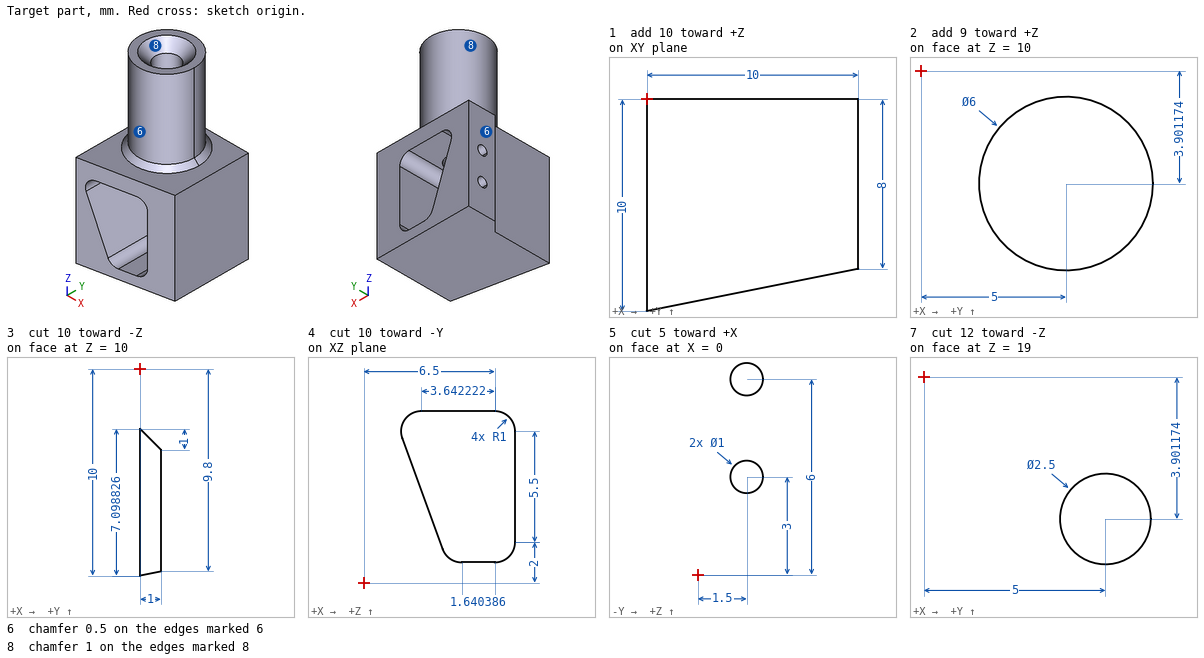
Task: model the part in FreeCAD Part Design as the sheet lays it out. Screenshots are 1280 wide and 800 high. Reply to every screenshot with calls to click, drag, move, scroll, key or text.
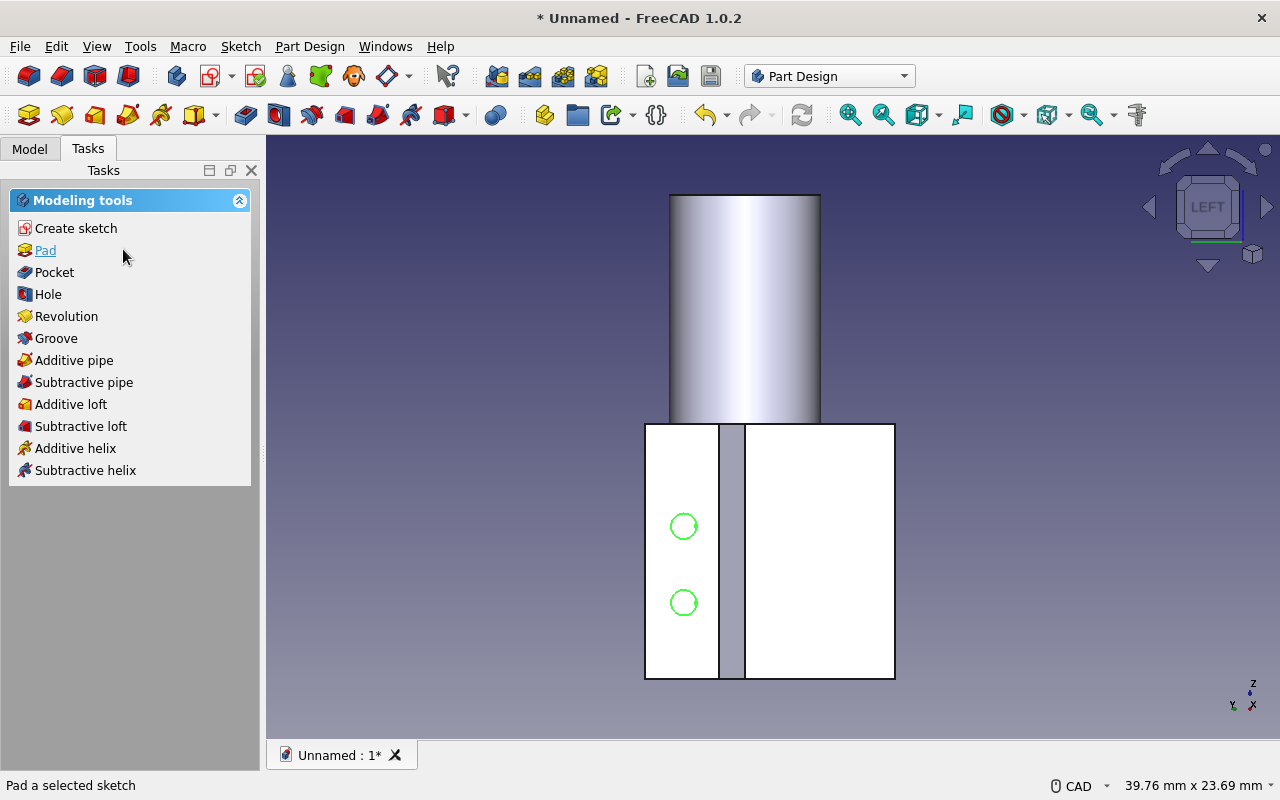
click(246, 116)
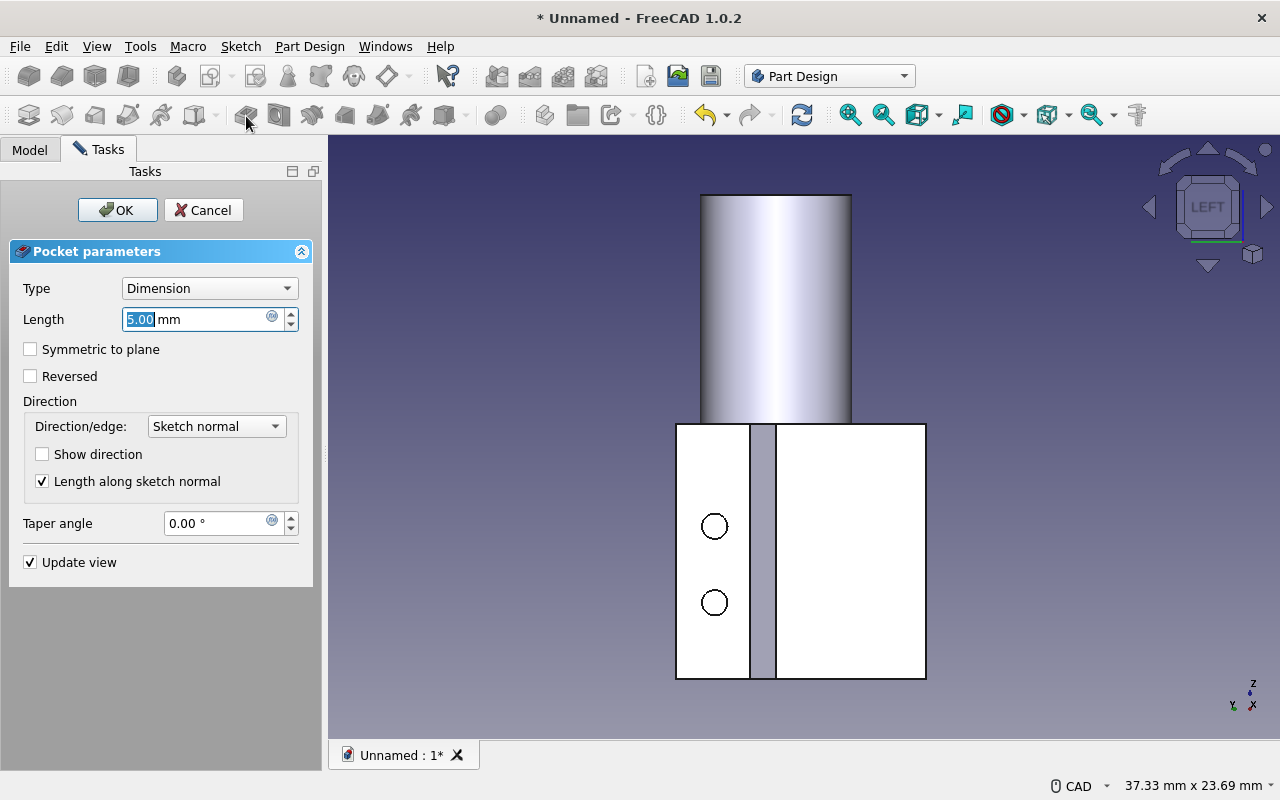
text(5)
key(Tab)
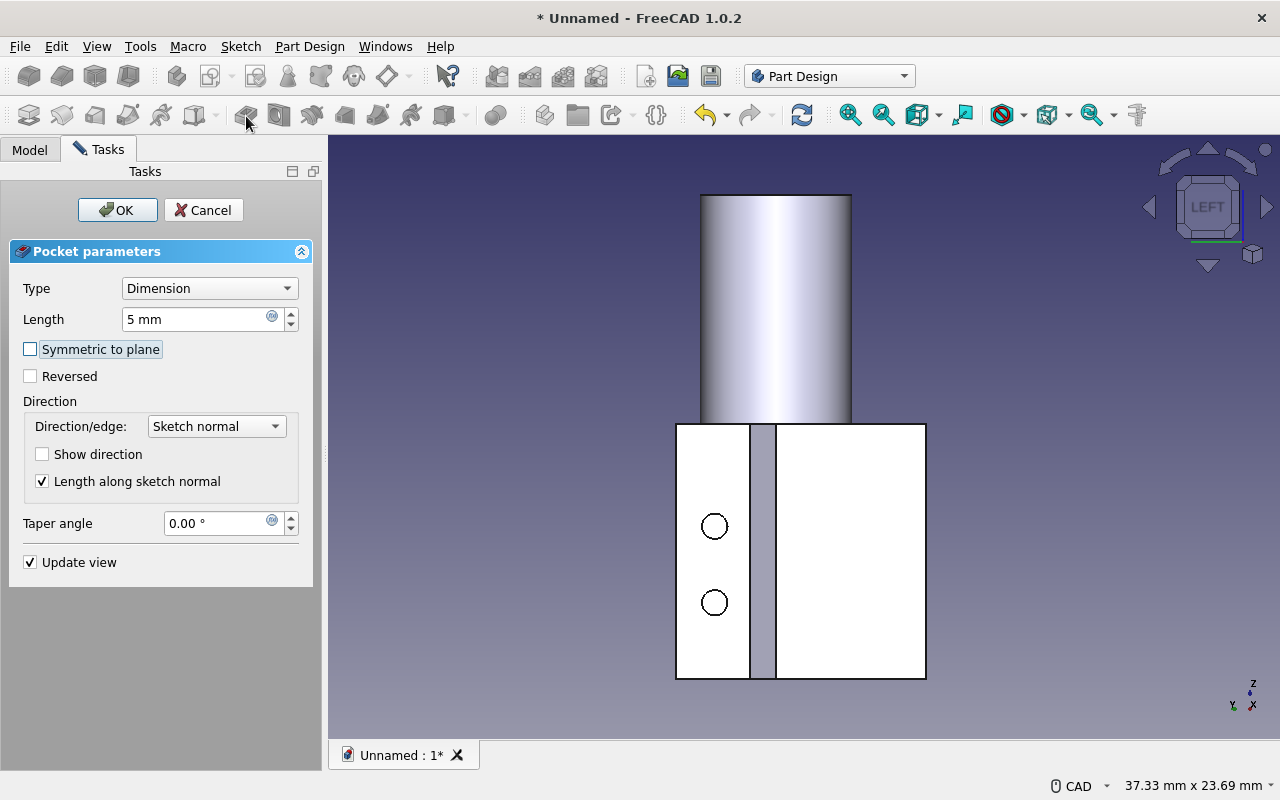
click(118, 210)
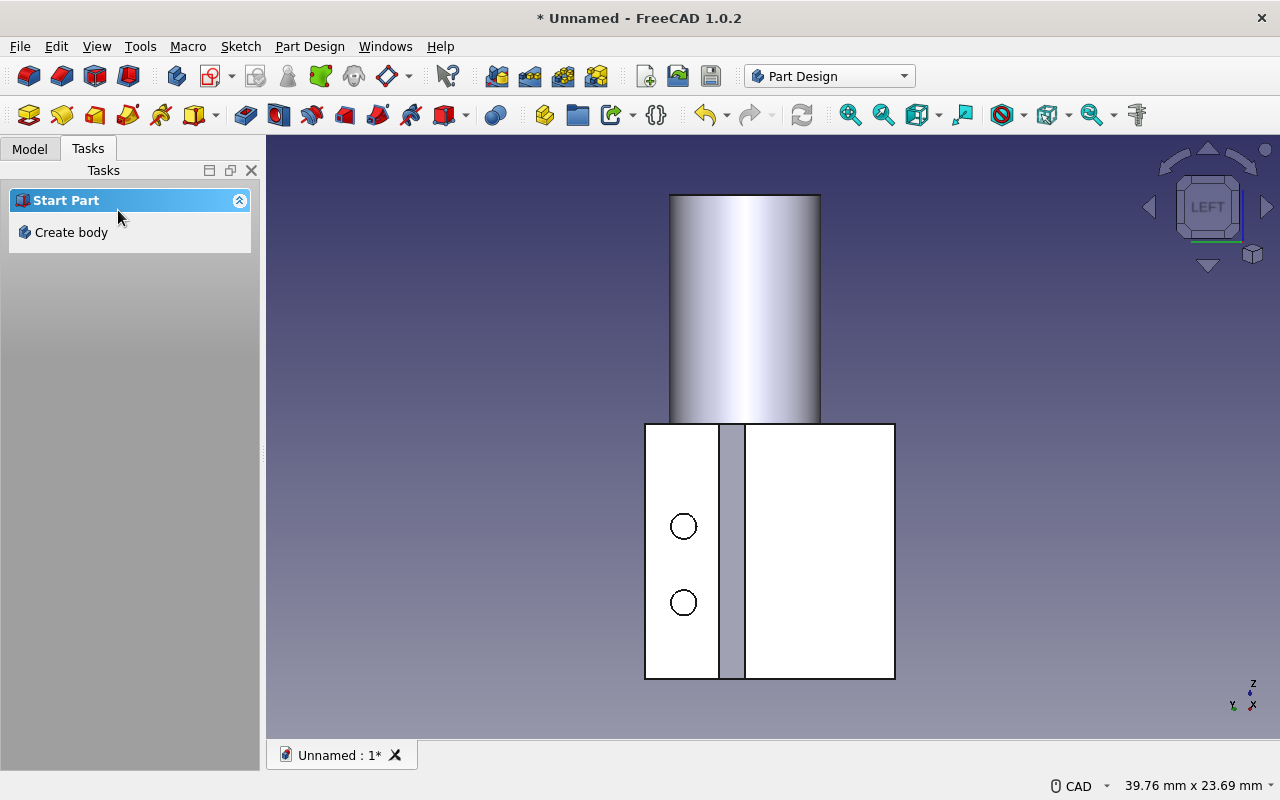
key(0)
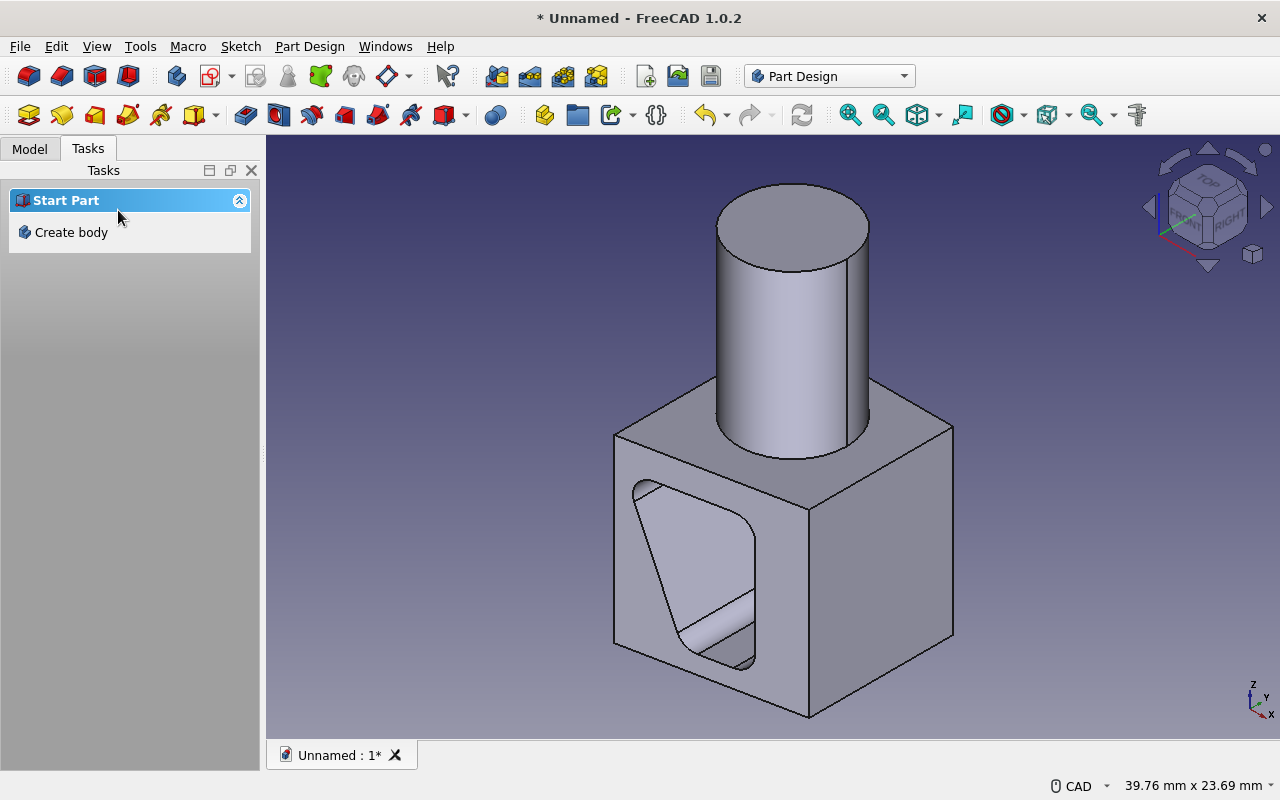
key(v)
key(f)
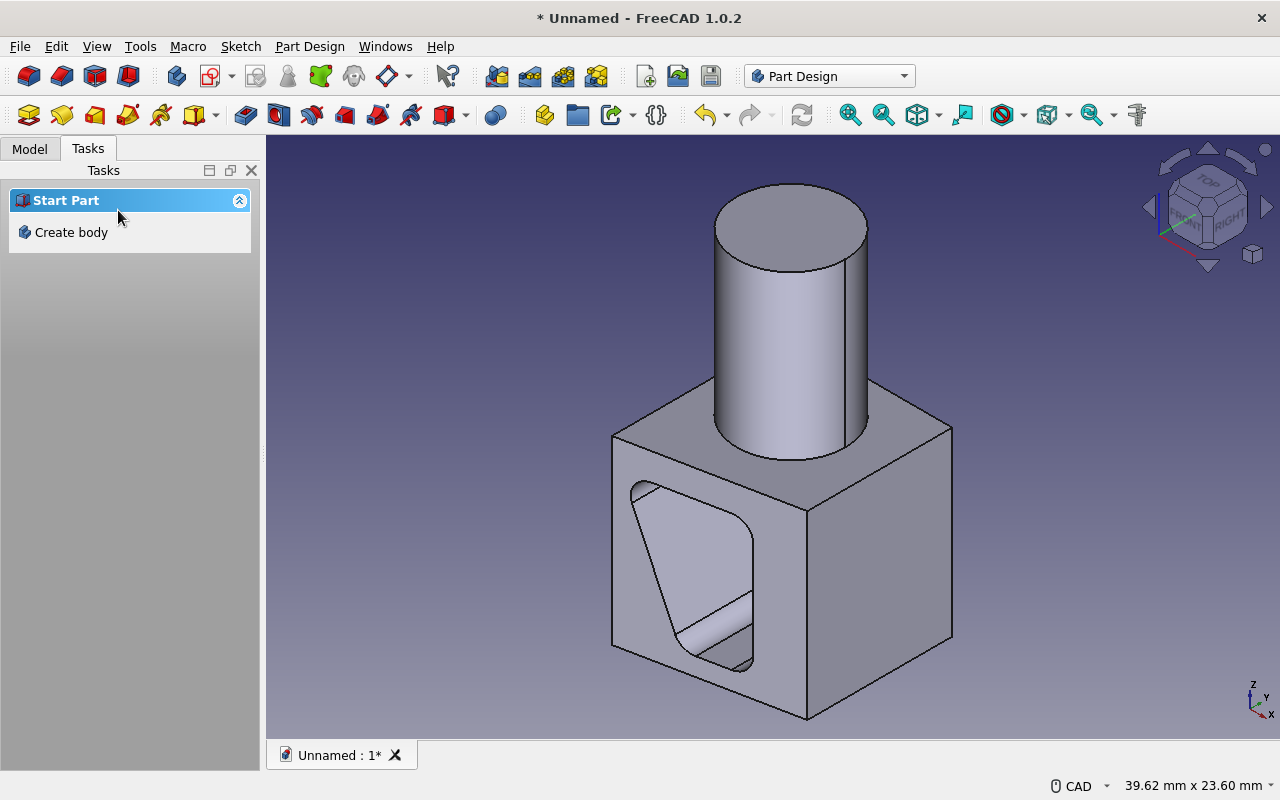
key(2)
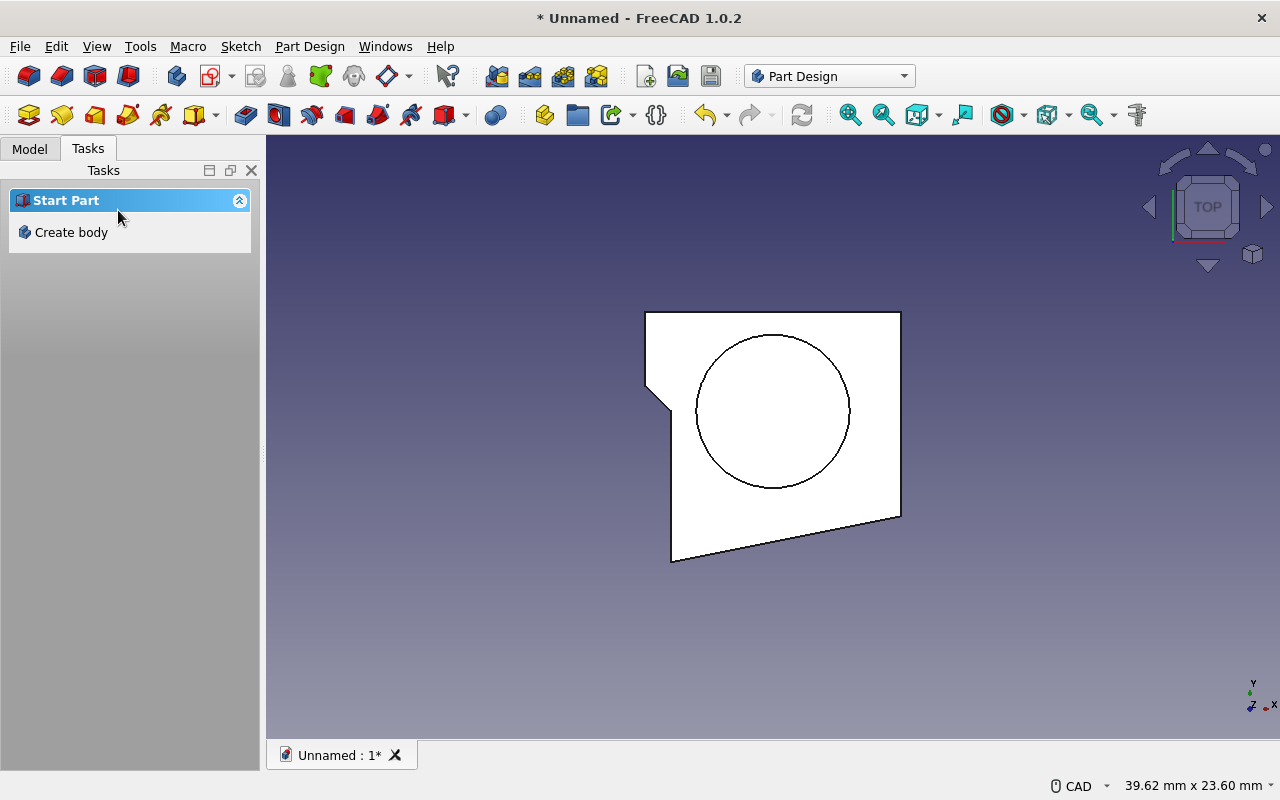
key(v)
key(f)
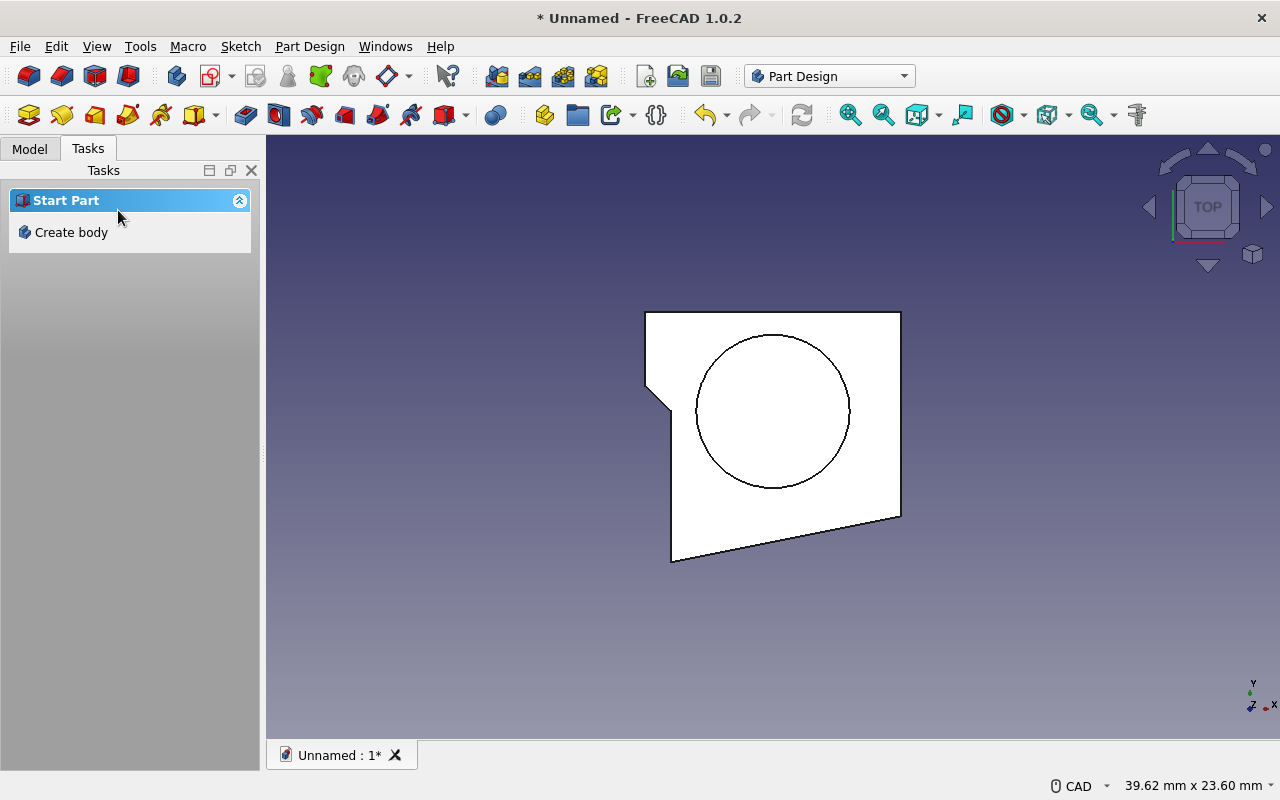
key(1)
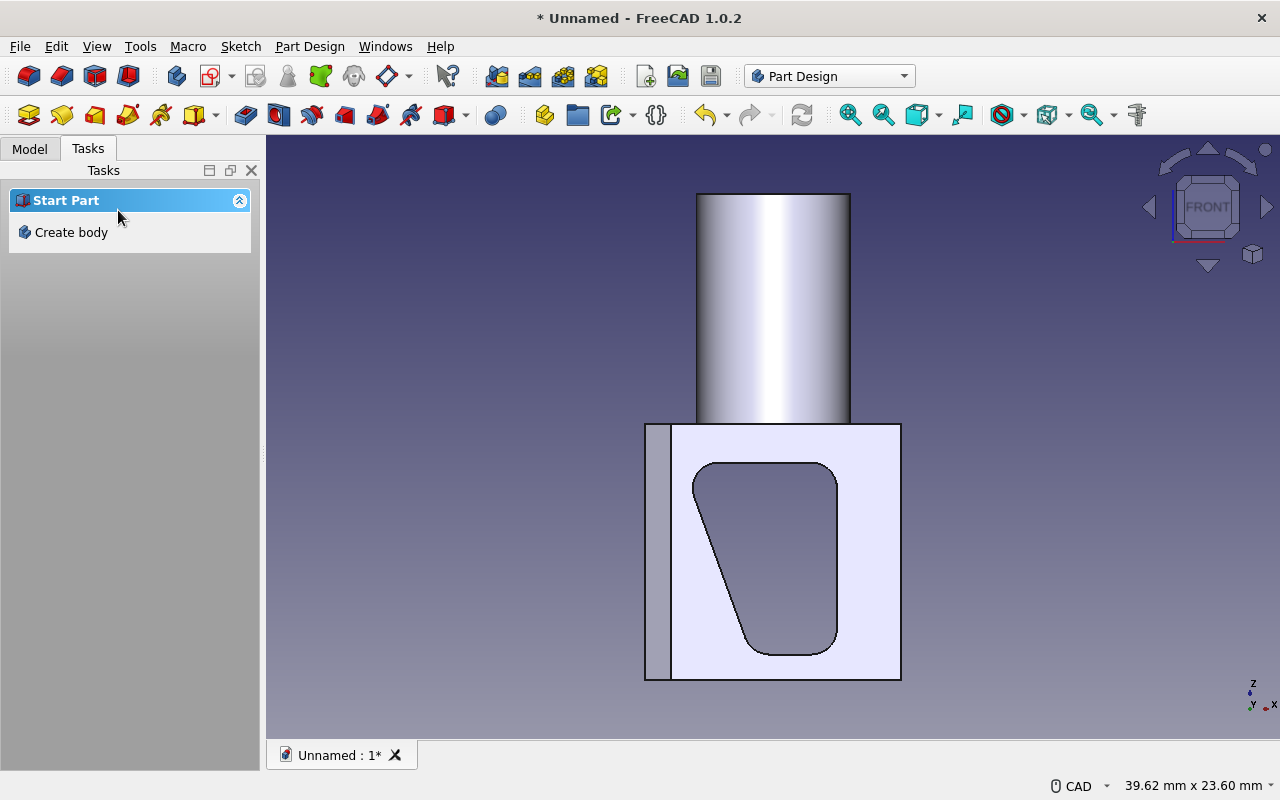
key(3)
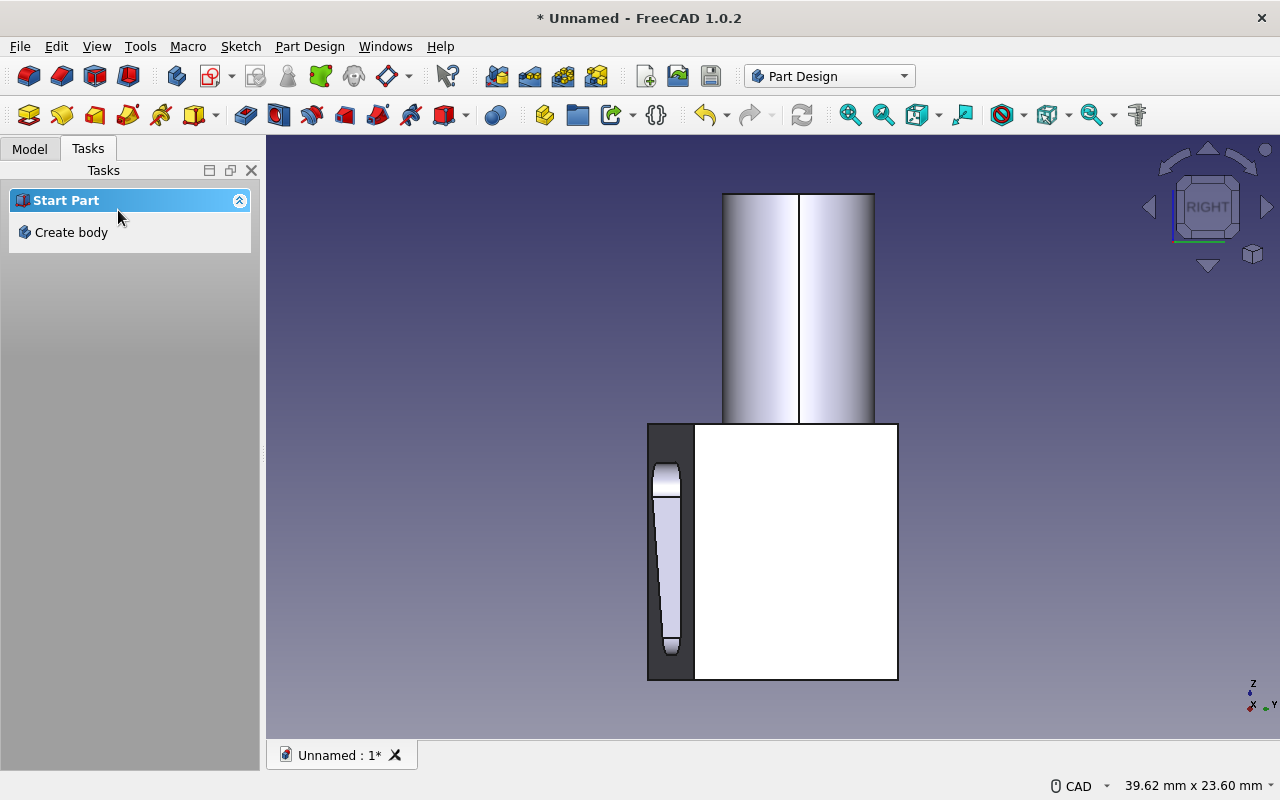
key(5)